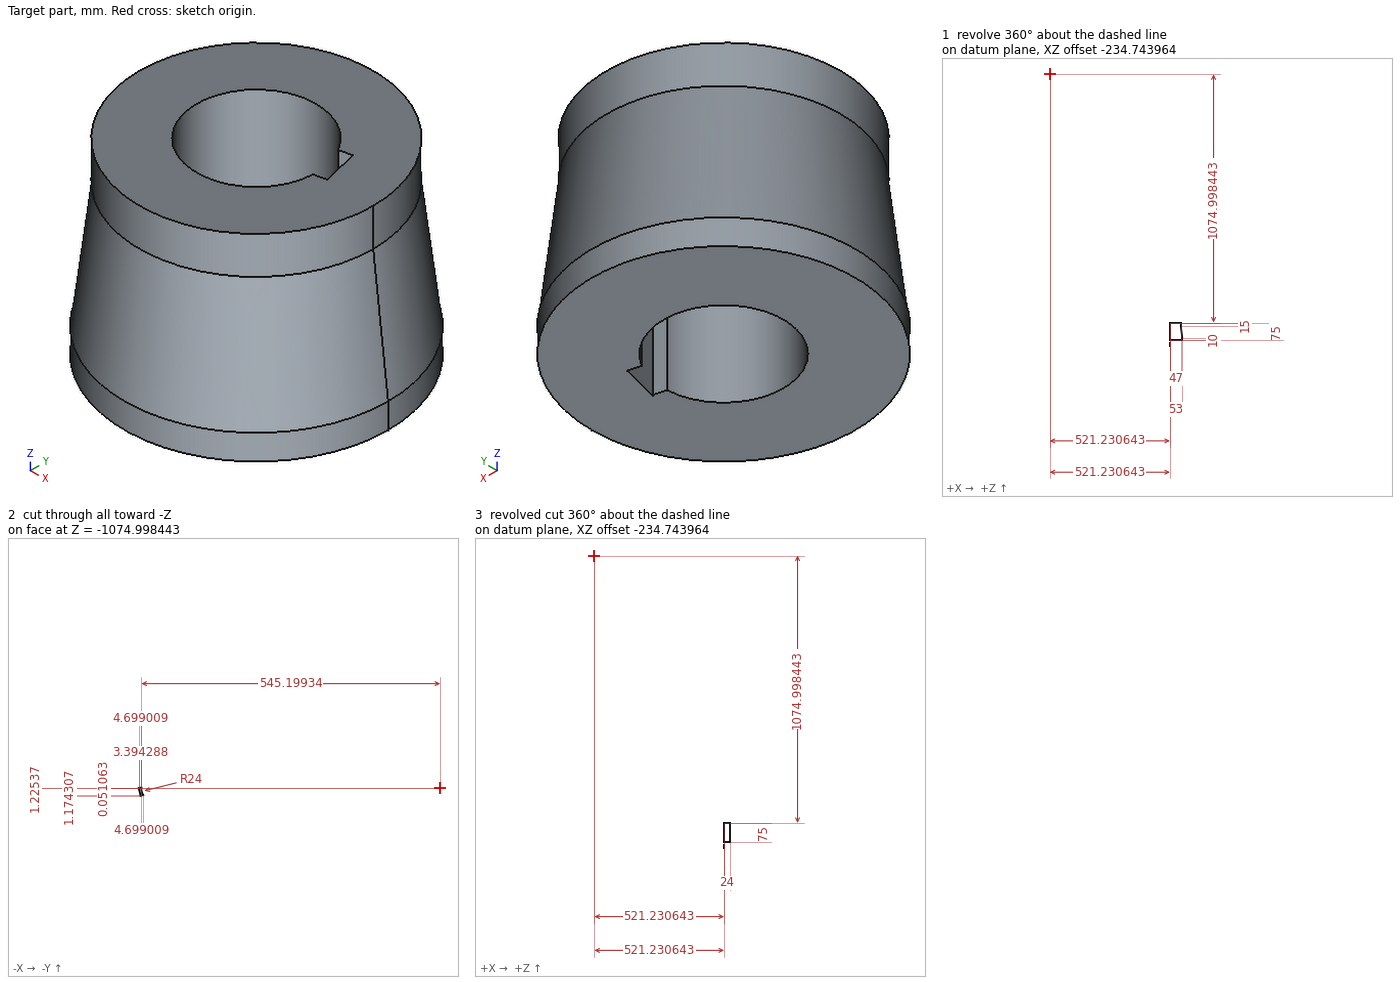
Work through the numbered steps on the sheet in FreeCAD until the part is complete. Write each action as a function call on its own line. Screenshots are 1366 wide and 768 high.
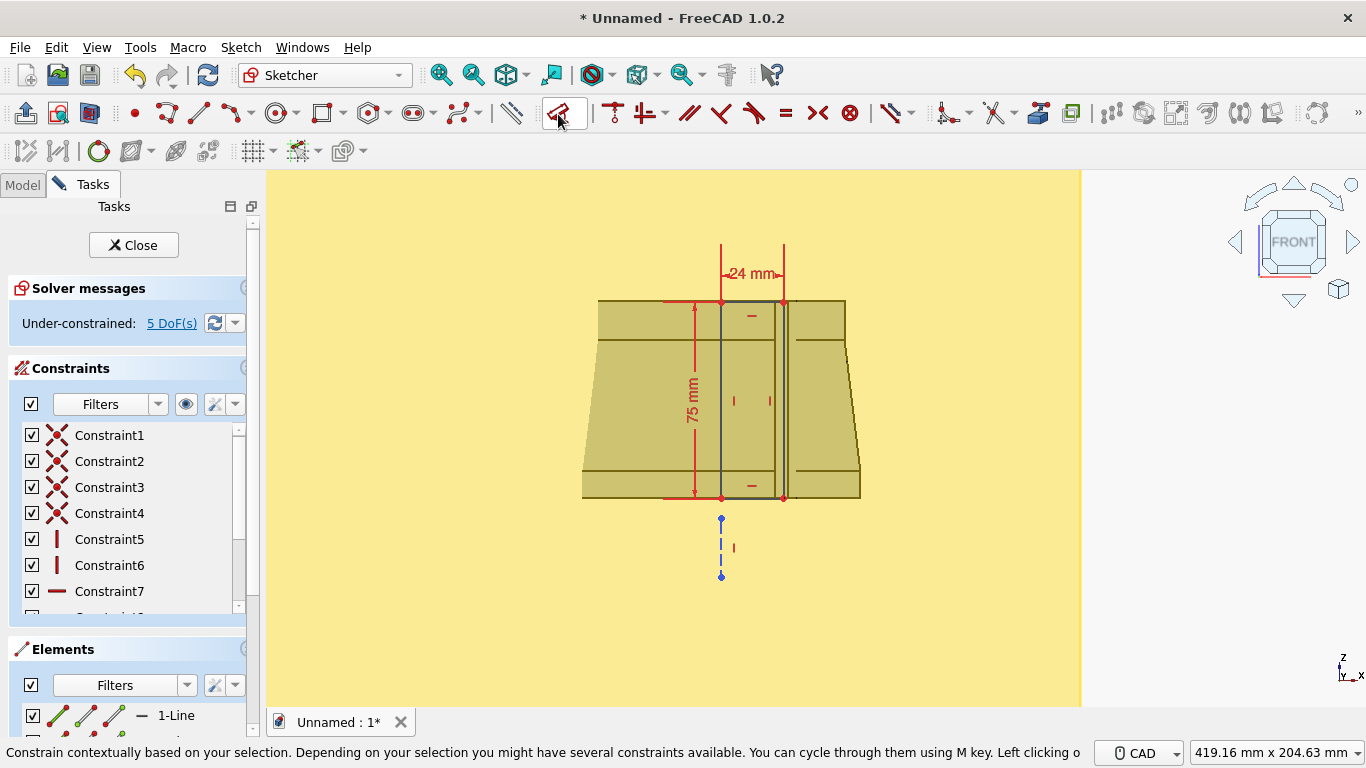
click(721, 302)
click(507, 336)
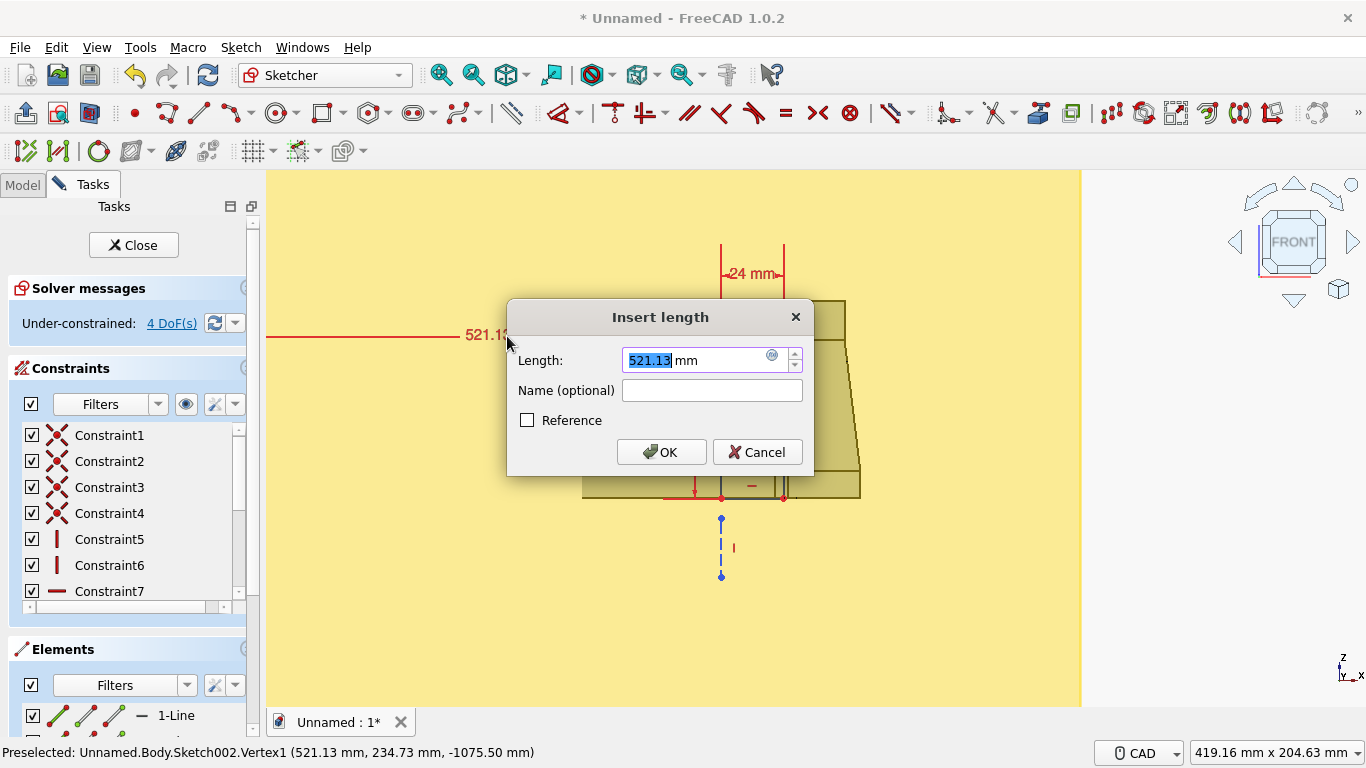
text(521.230643)
key(Return)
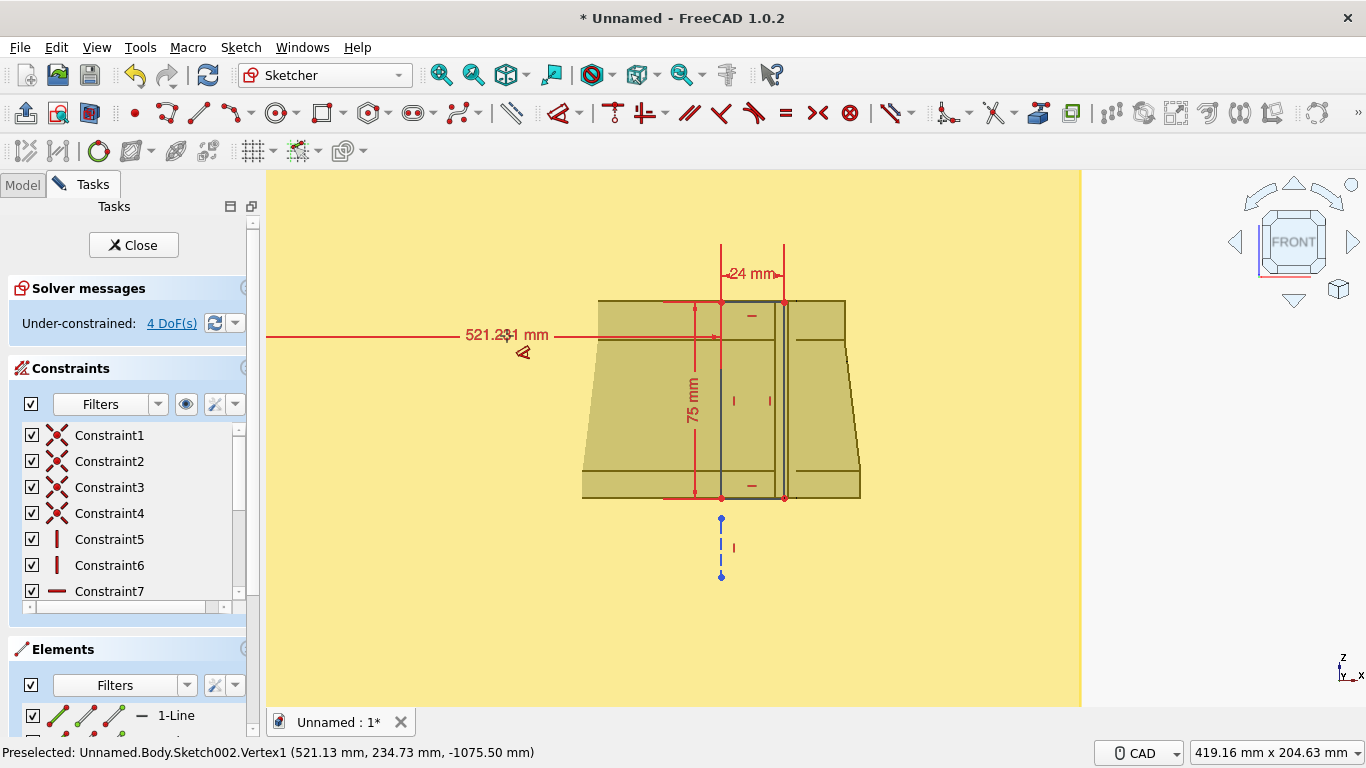
click(721, 518)
click(507, 552)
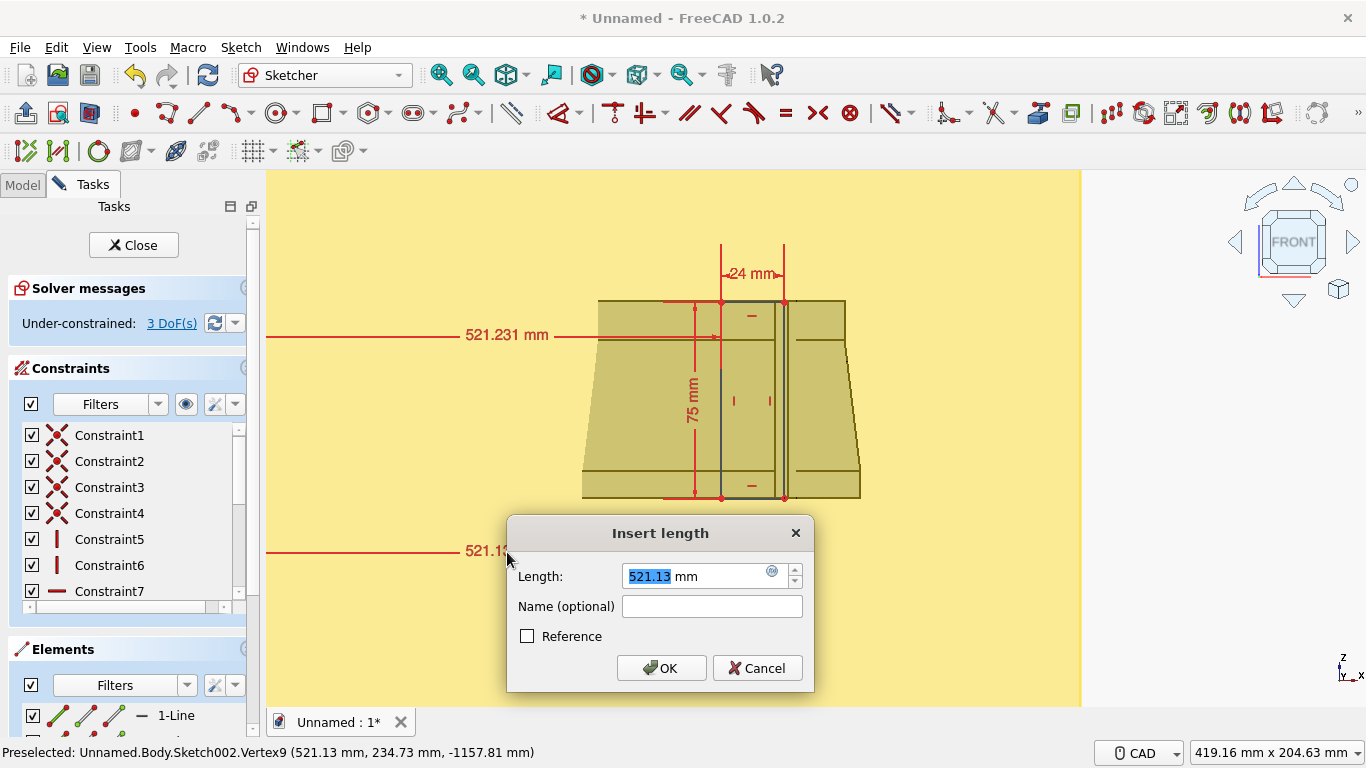
text(521.230643)
key(Return)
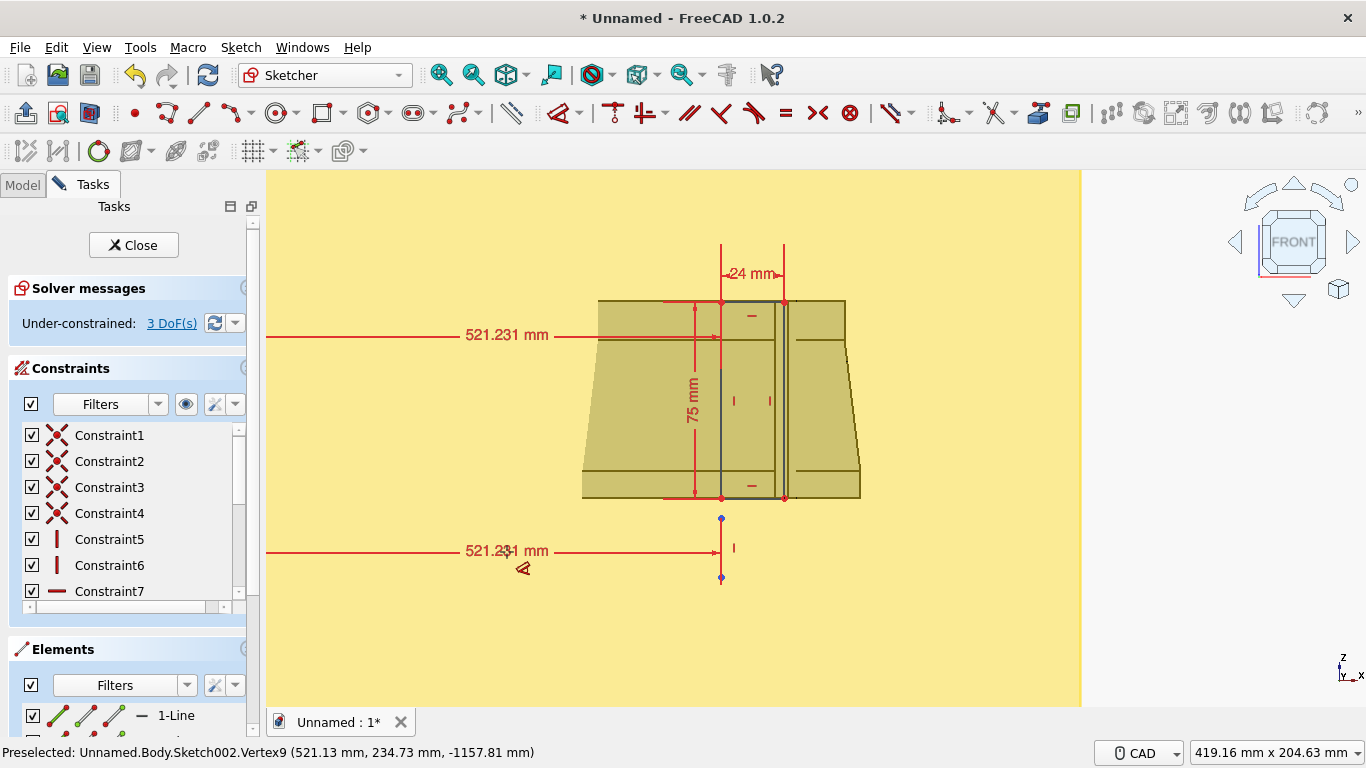
click(721, 302)
click(755, 250)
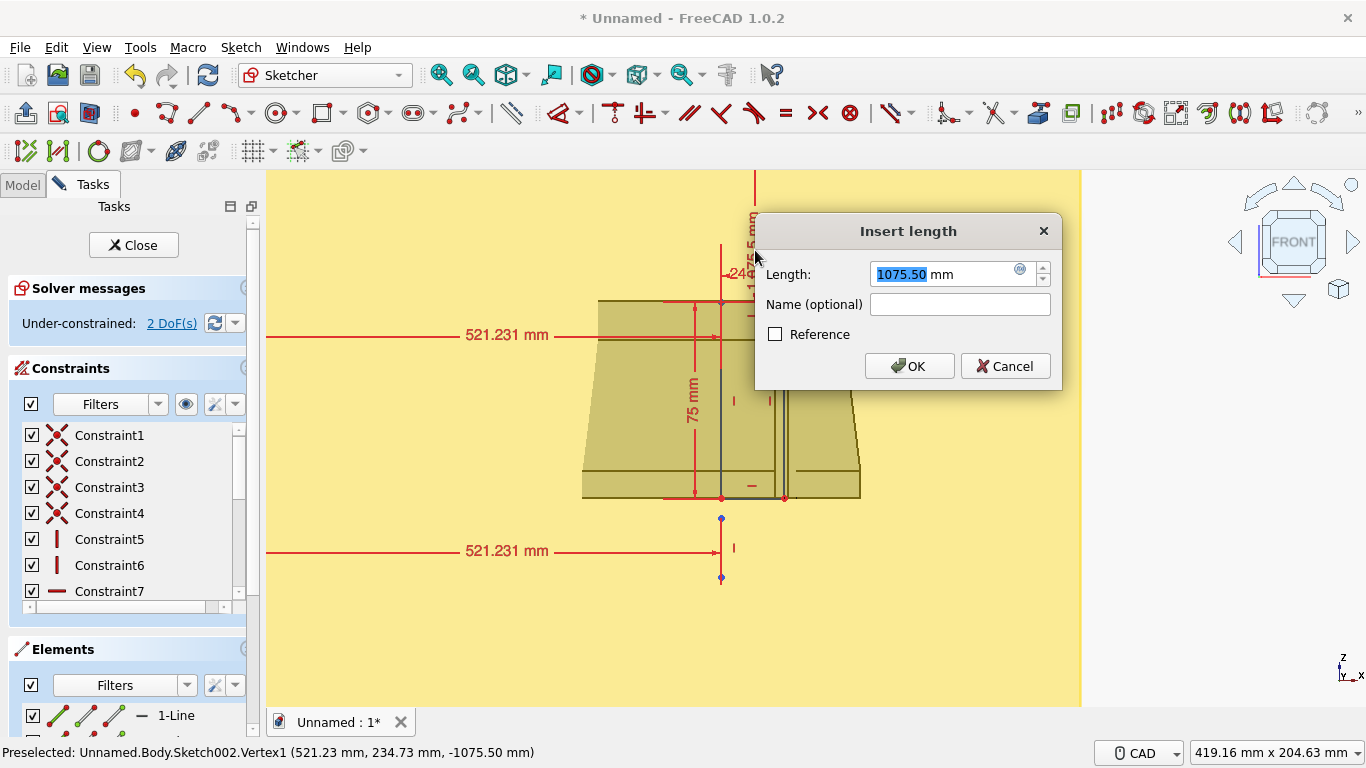
text(1074.998443)
key(Return)
key(Escape)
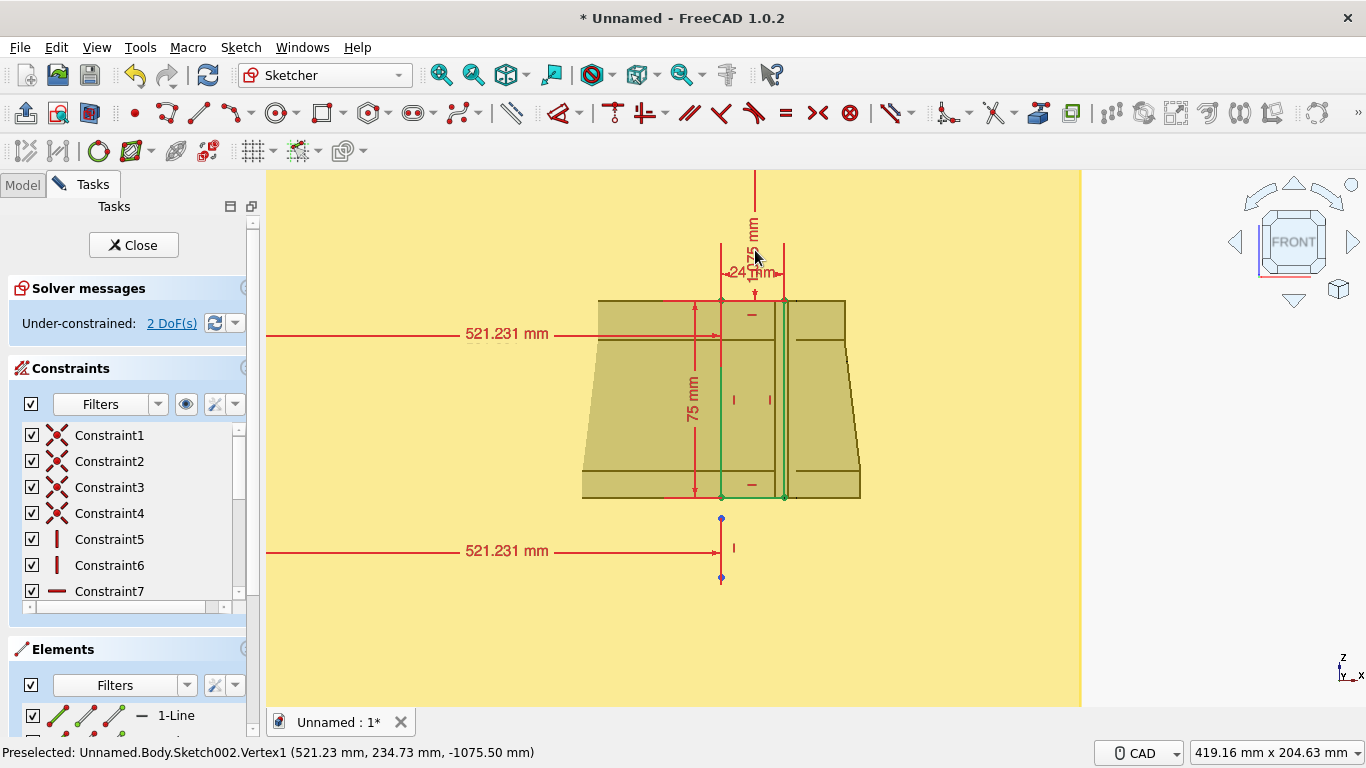
click(134, 245)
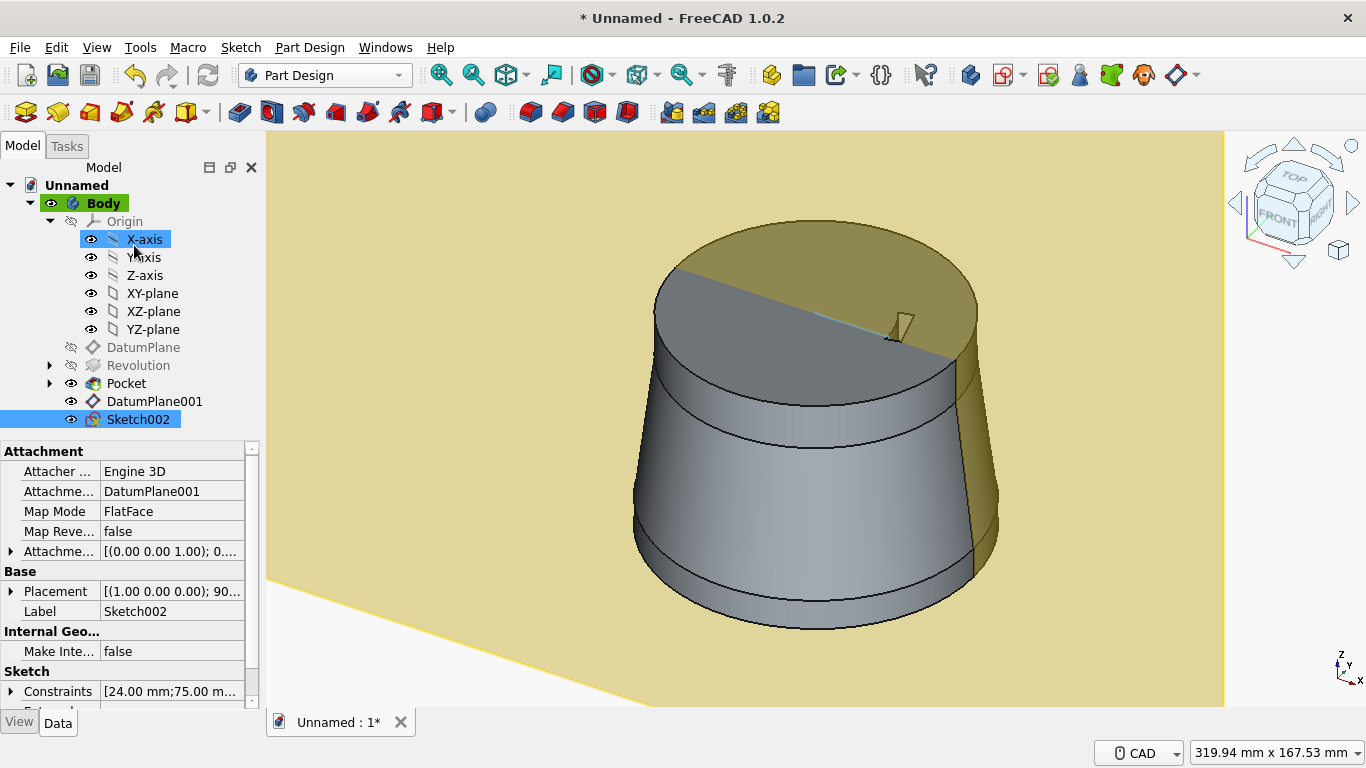
click(304, 112)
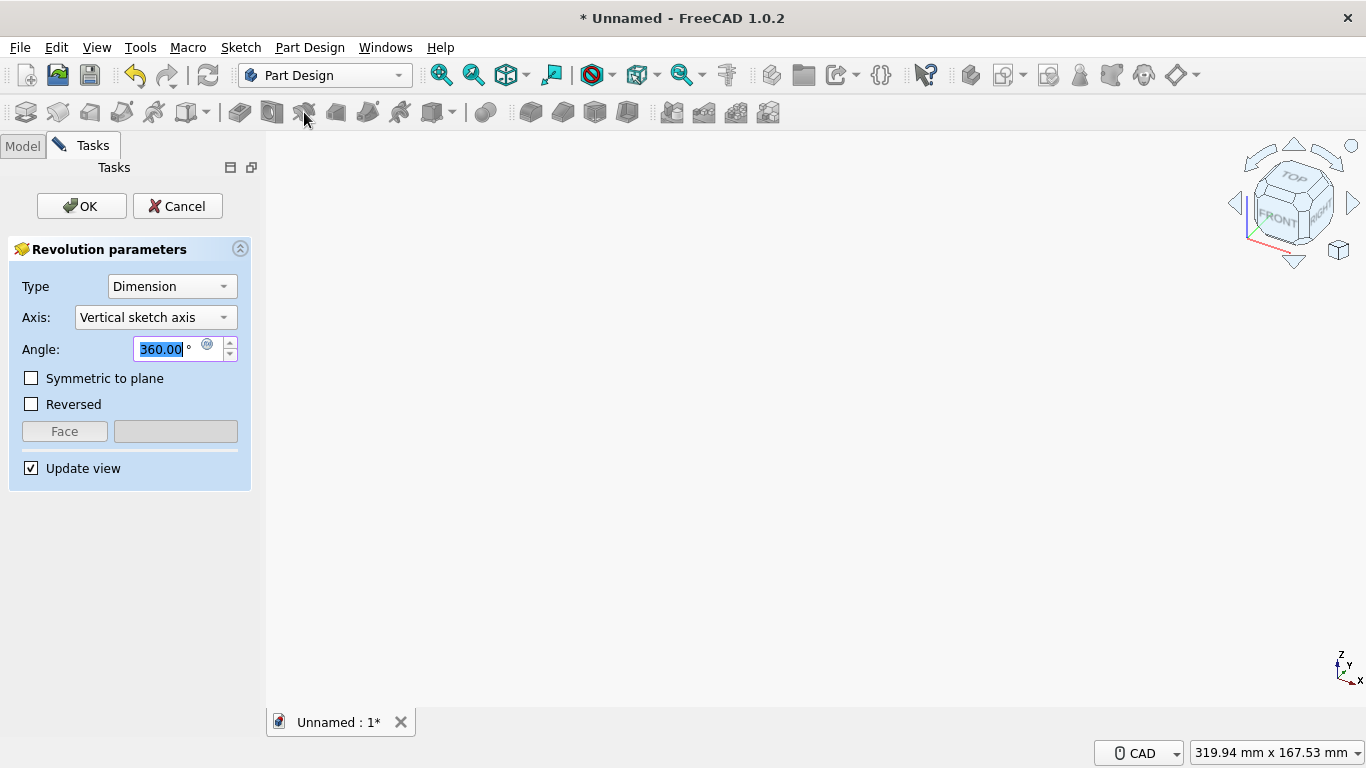
click(156, 318)